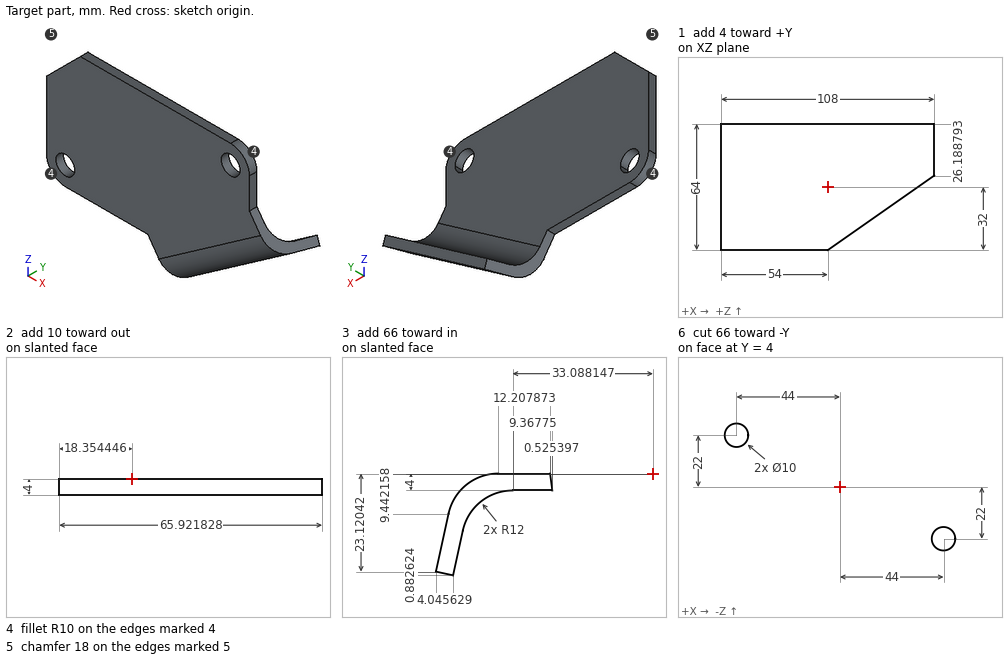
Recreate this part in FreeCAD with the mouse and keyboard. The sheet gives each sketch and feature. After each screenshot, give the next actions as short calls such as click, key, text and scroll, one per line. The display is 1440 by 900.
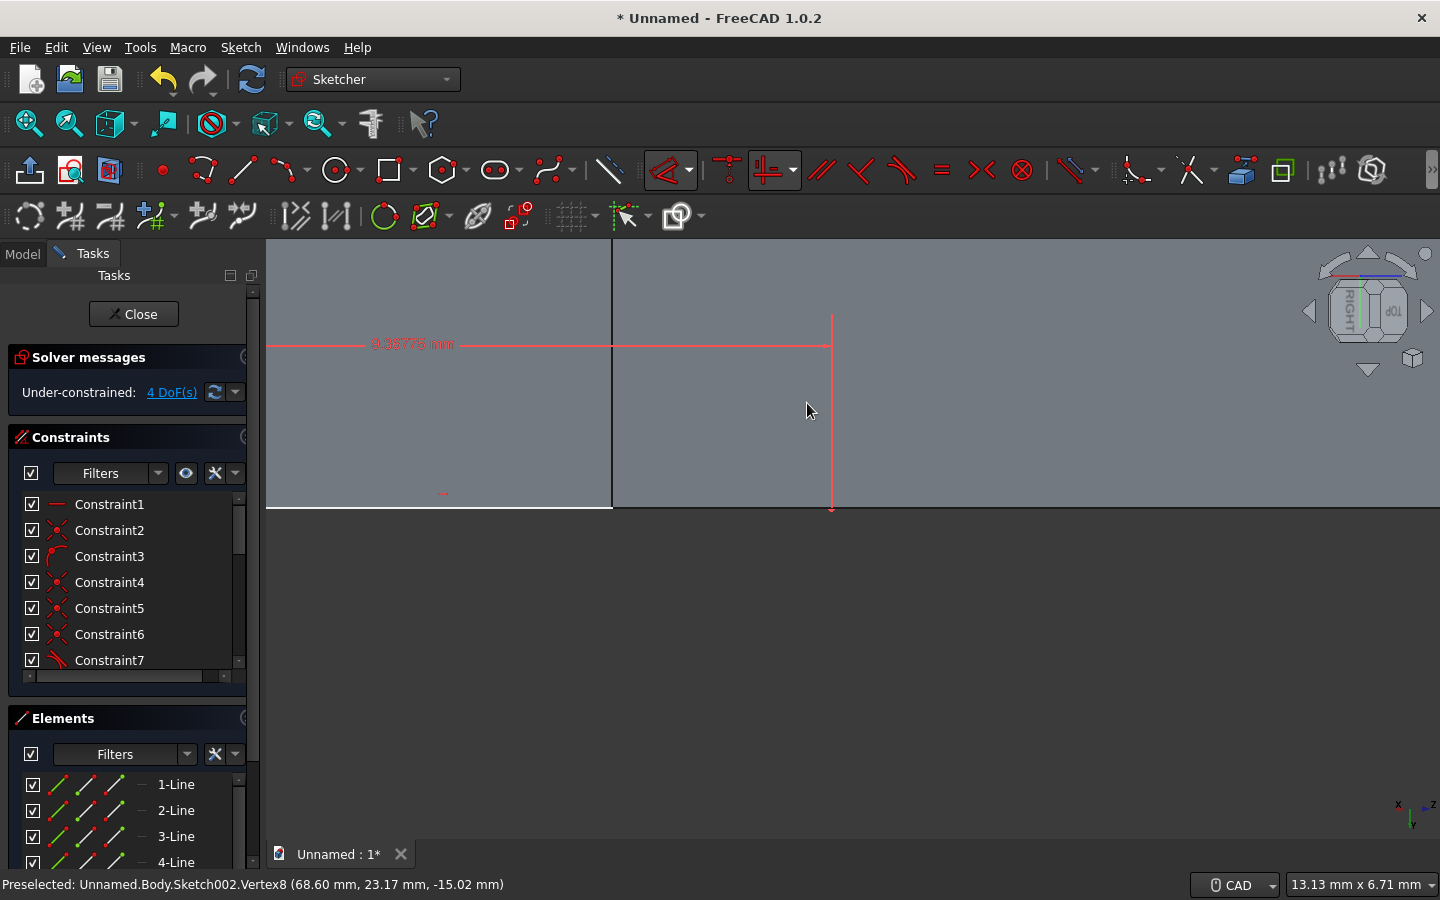
click(806, 401)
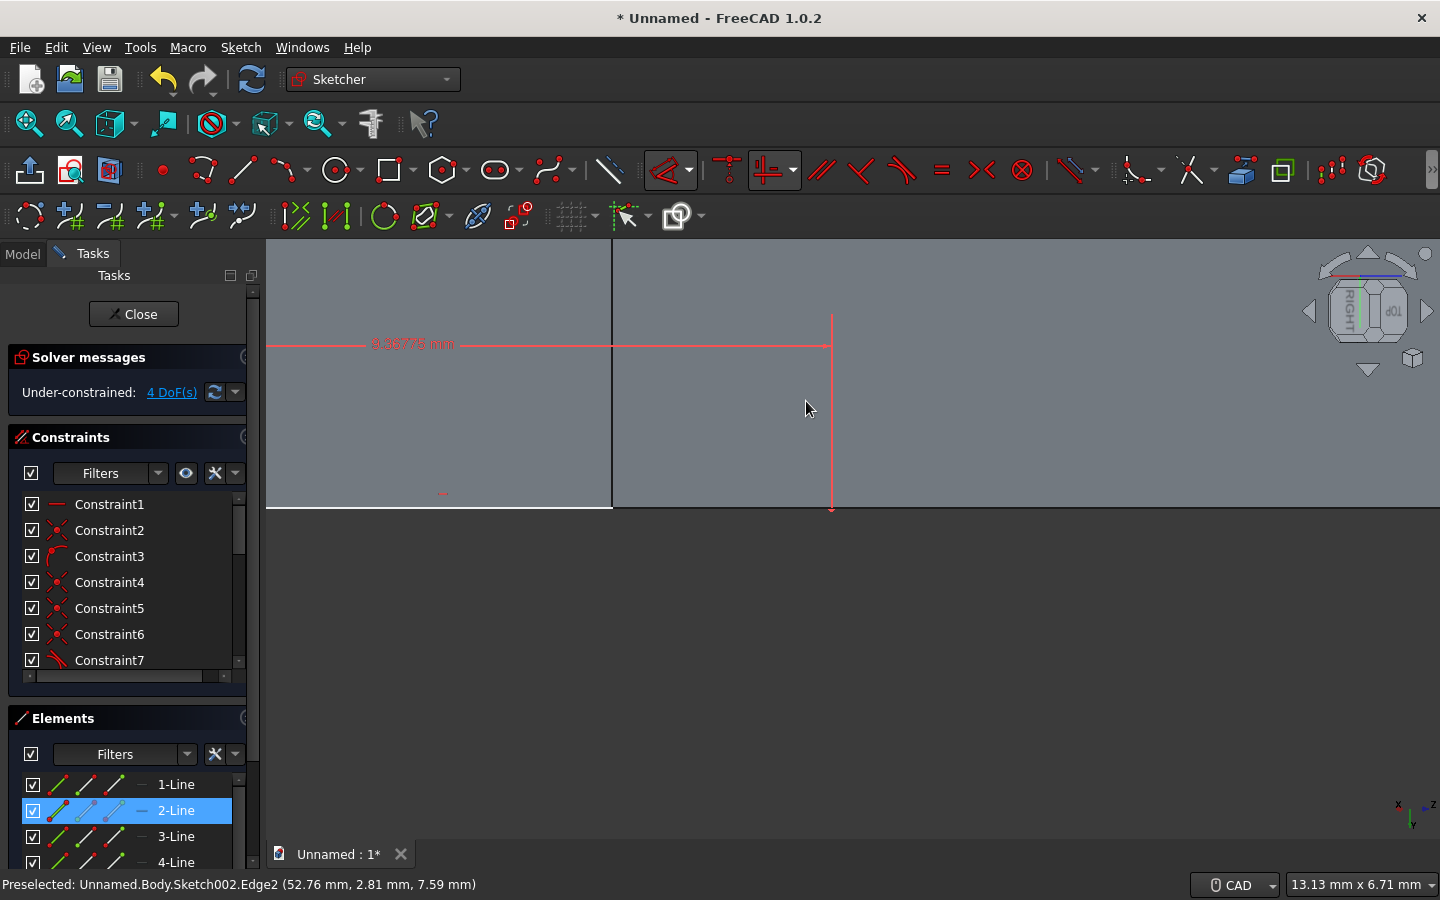
key(l)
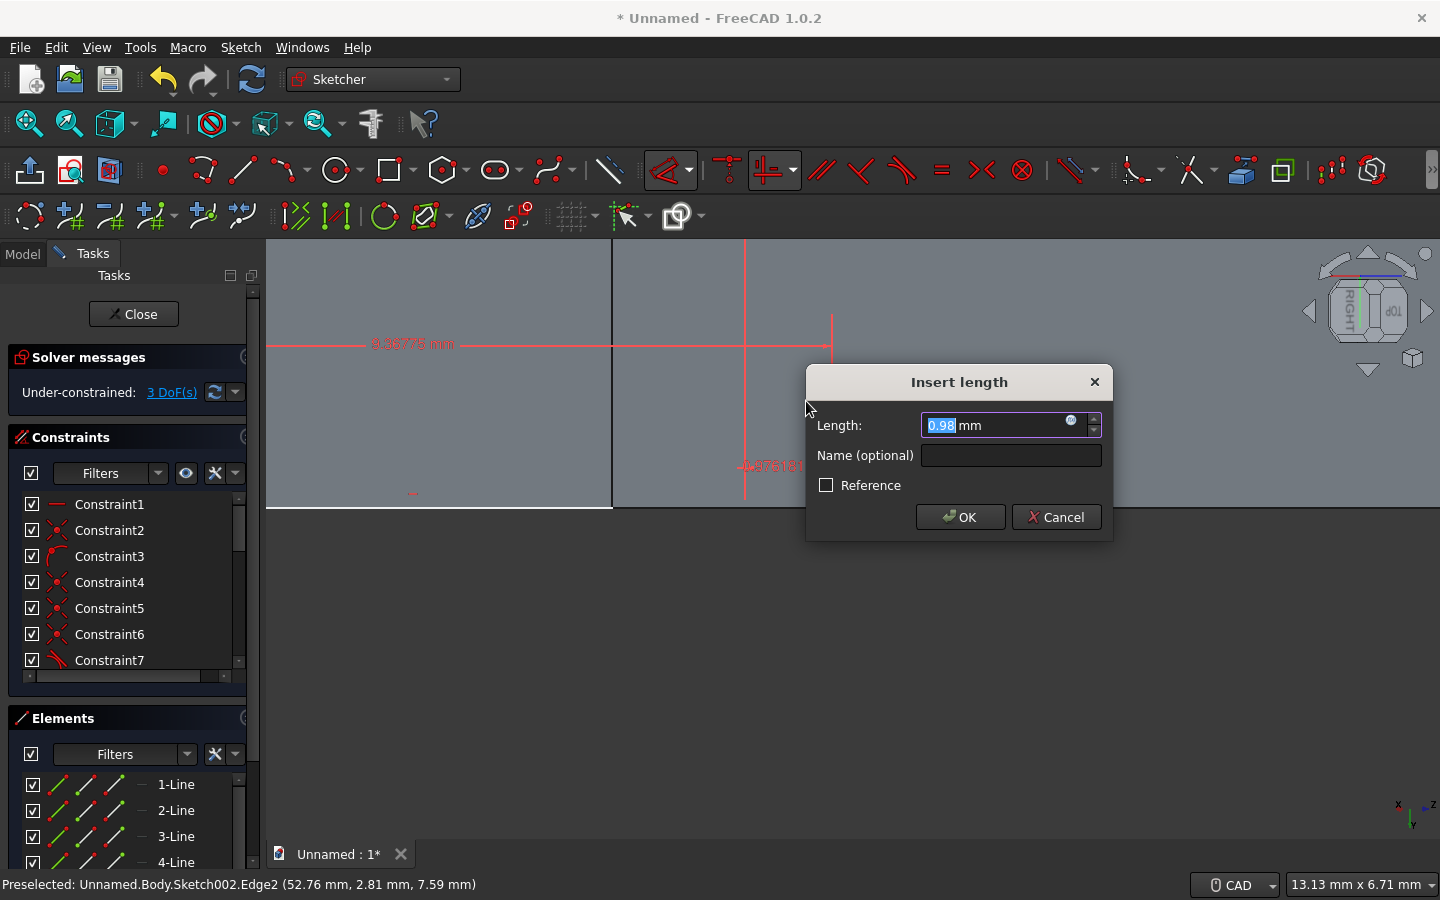
text(0.525397)
key(Return)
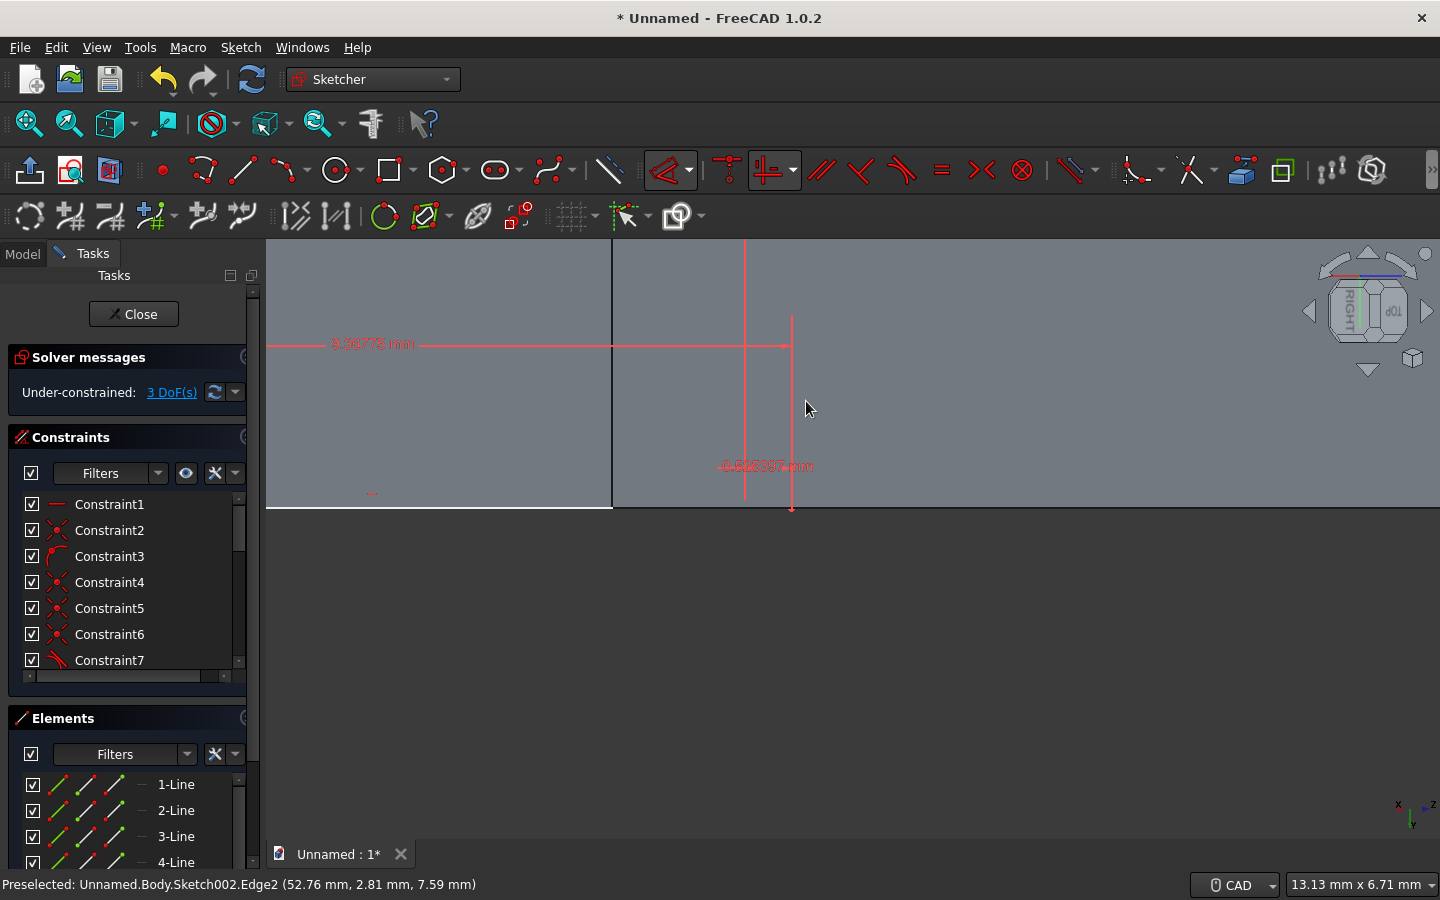
scroll(807, 403, down, 9)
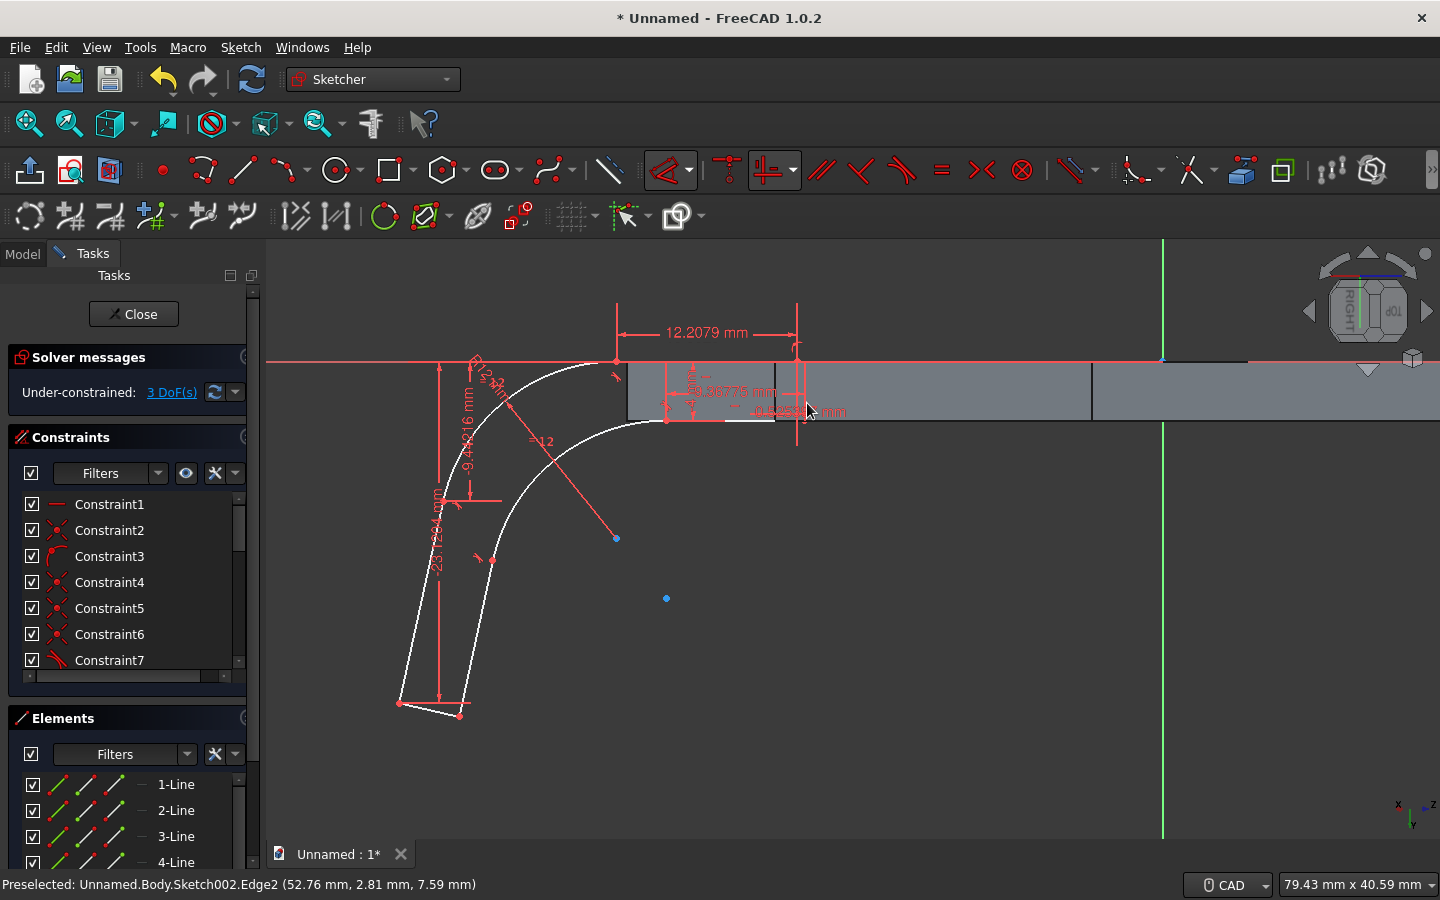
click(417, 707)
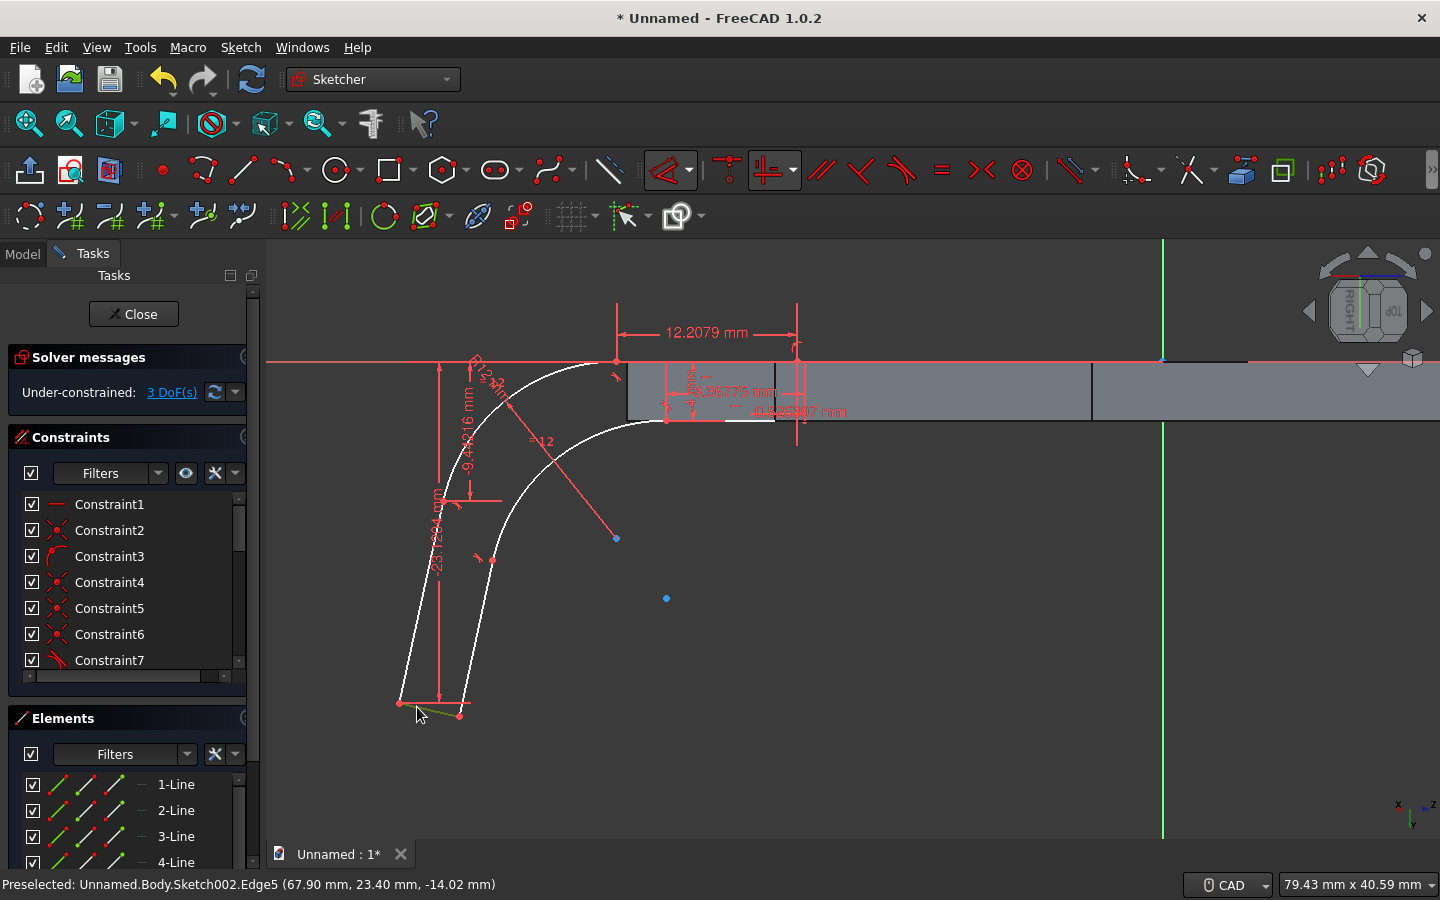
key(l)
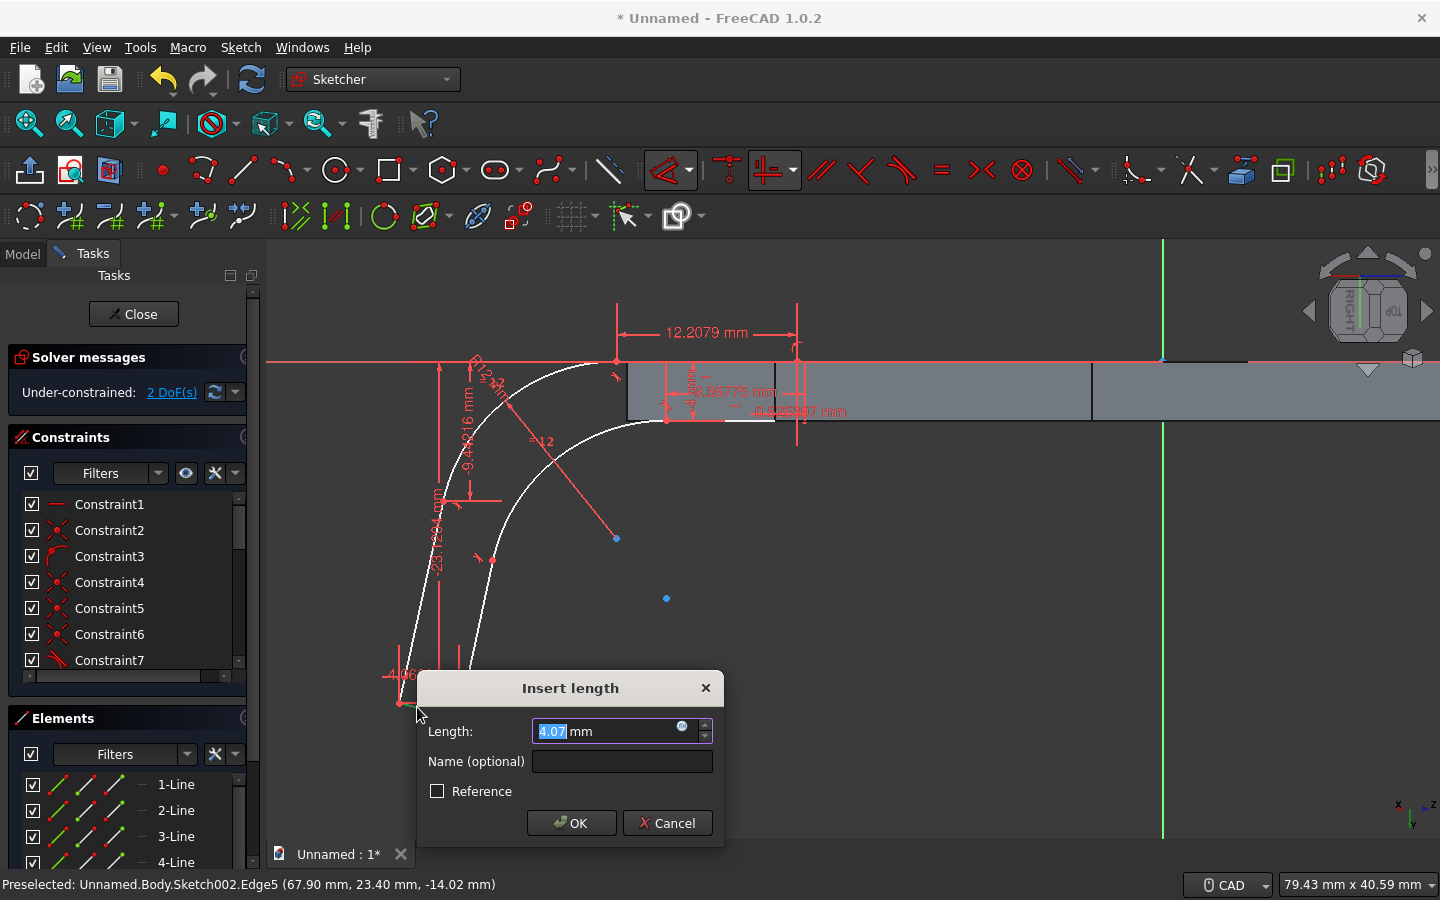
text(4.045629)
key(Return)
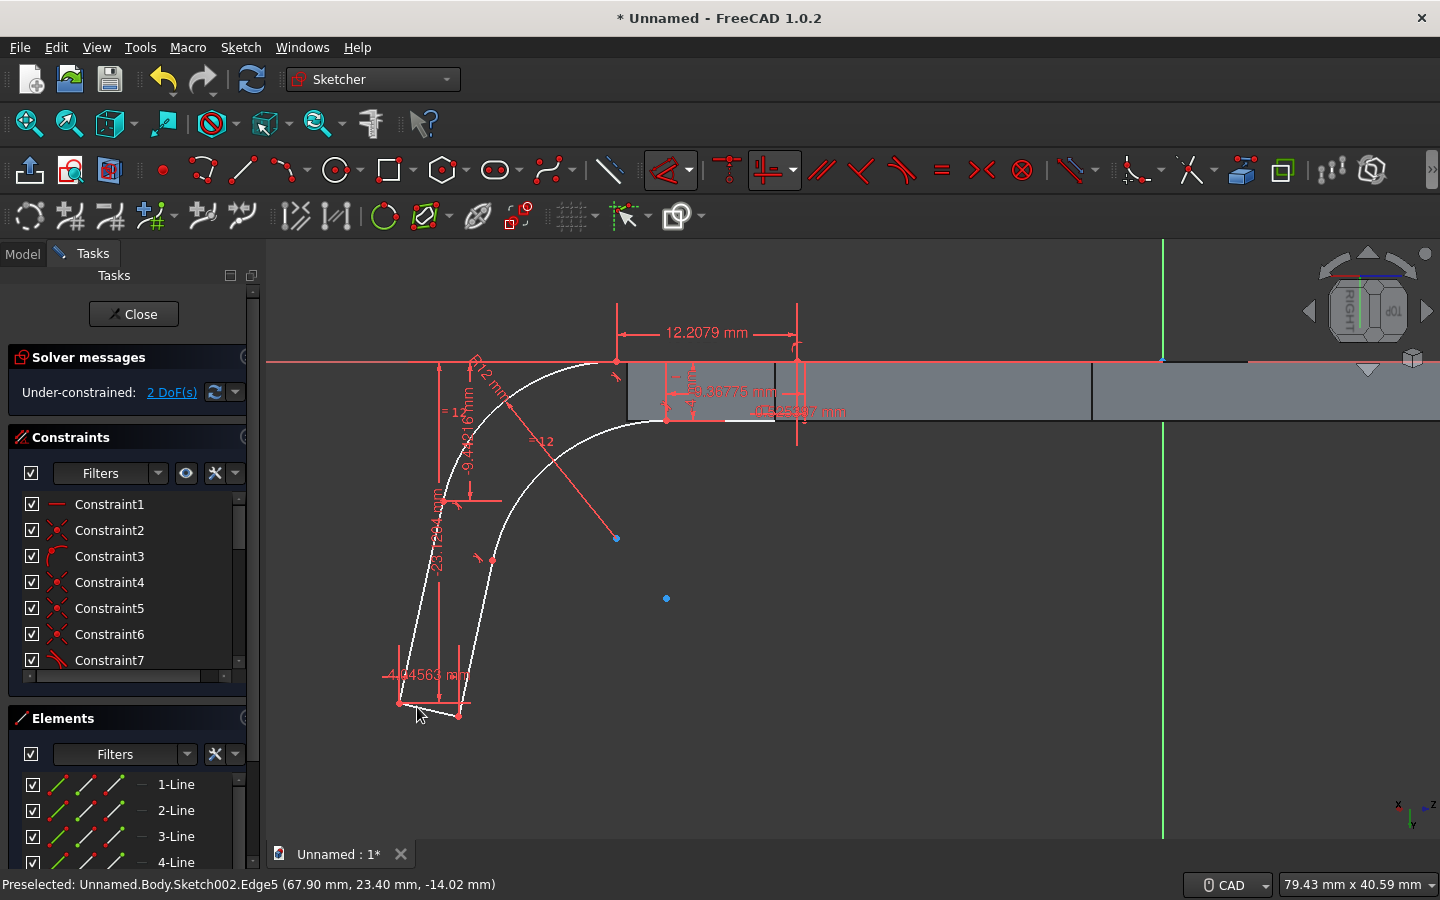
scroll(417, 707, up, 6)